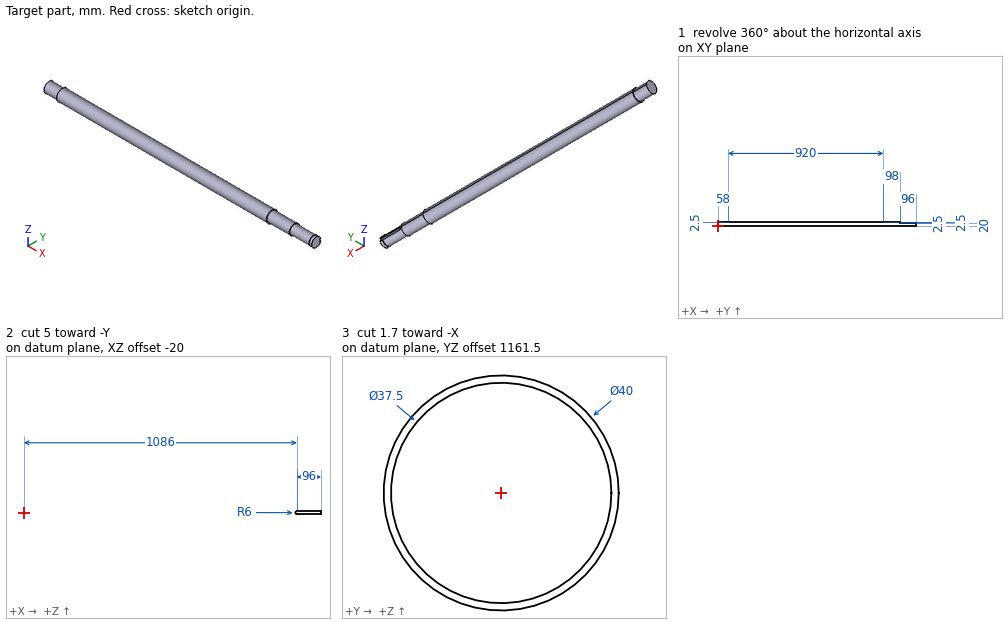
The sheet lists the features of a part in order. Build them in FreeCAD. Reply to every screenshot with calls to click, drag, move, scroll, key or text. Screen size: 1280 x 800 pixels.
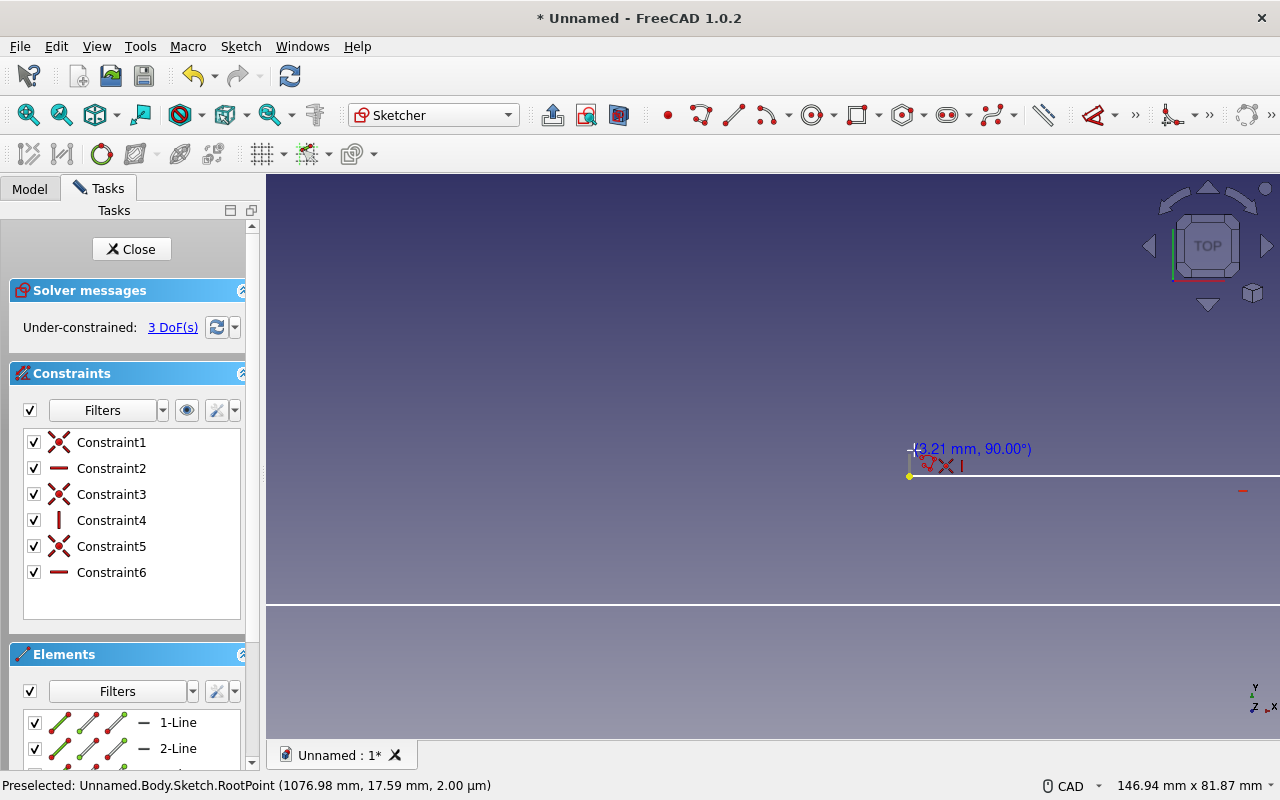
click(910, 450)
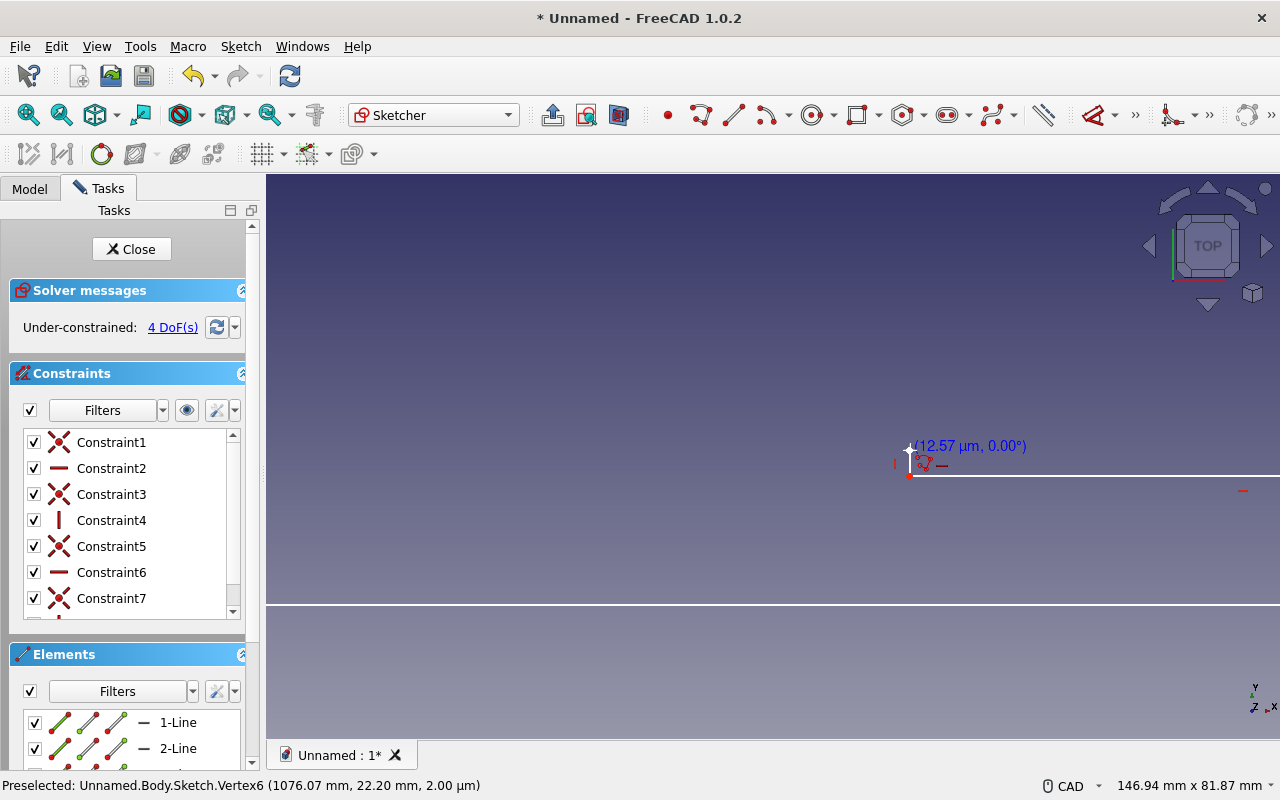
scroll(959, 451, down, 13)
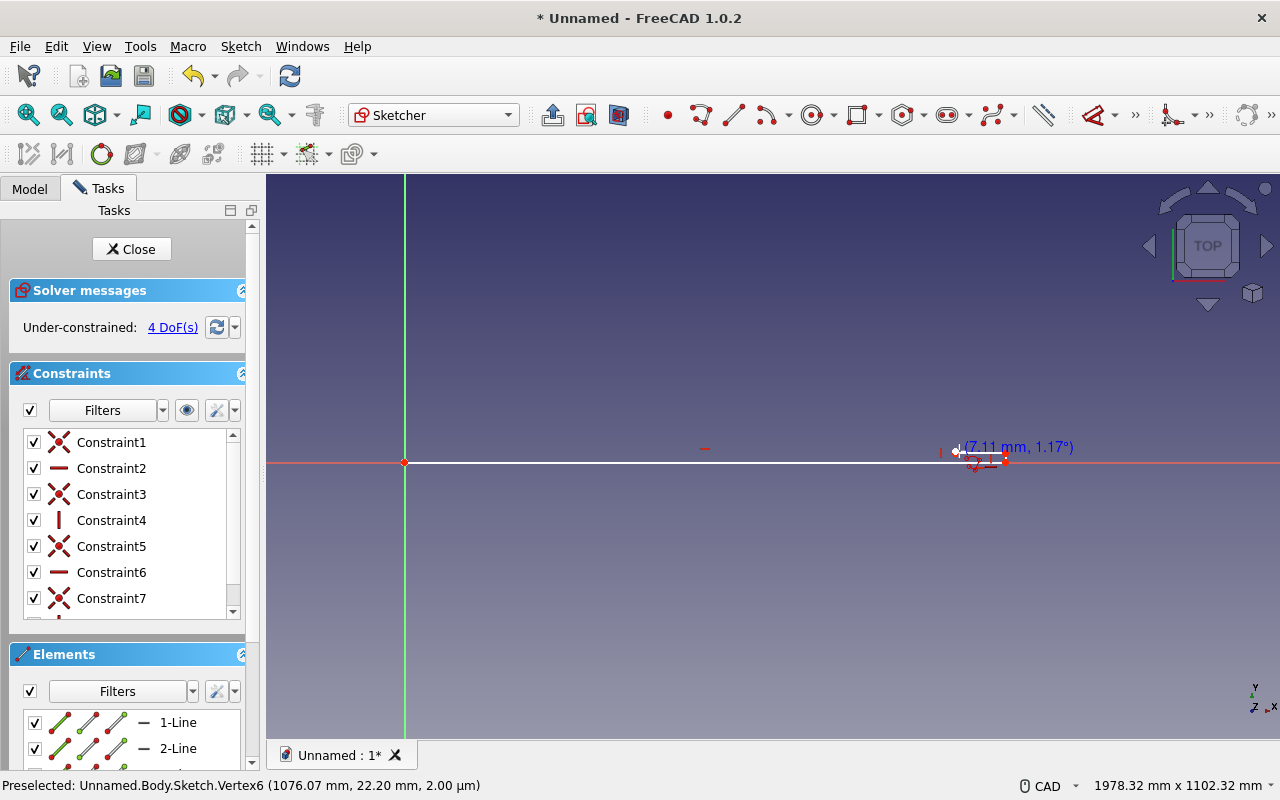
scroll(906, 451, up, 2)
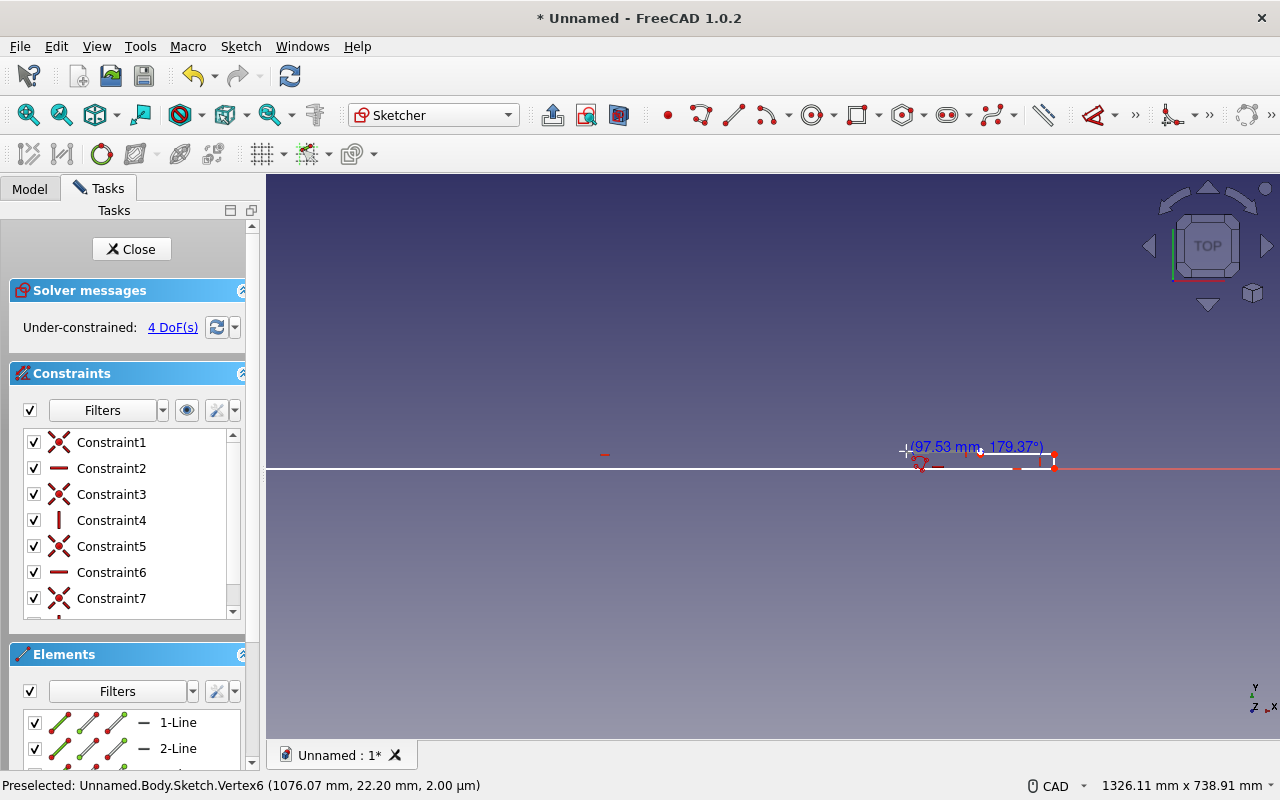
click(905, 451)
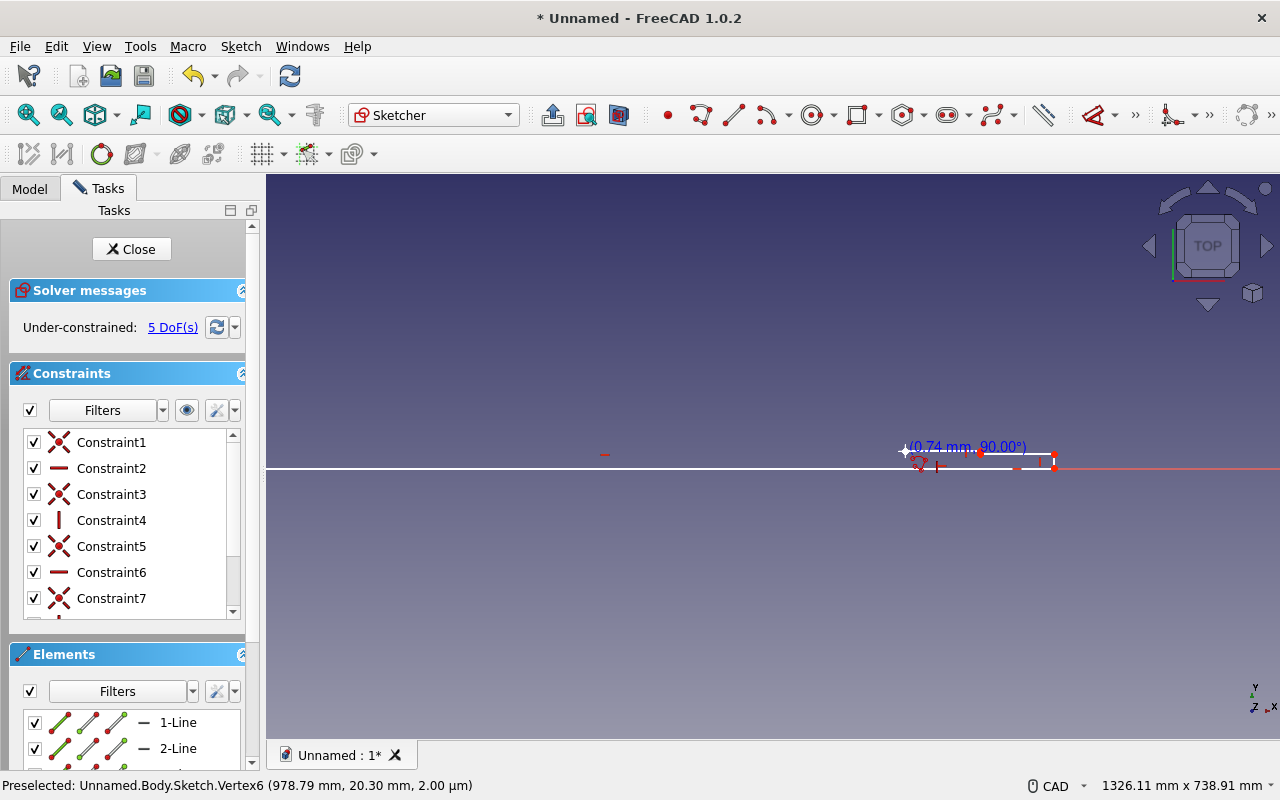
scroll(905, 449, up, 11)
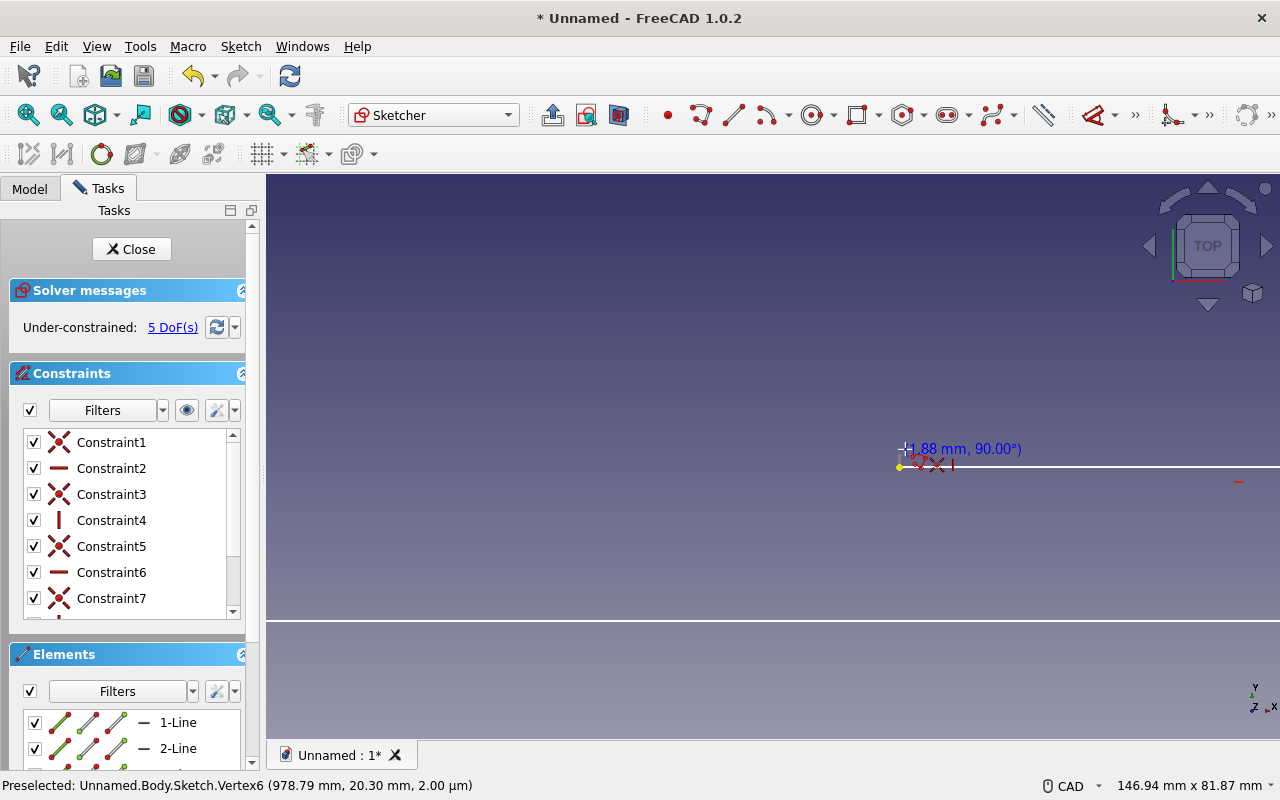
click(900, 449)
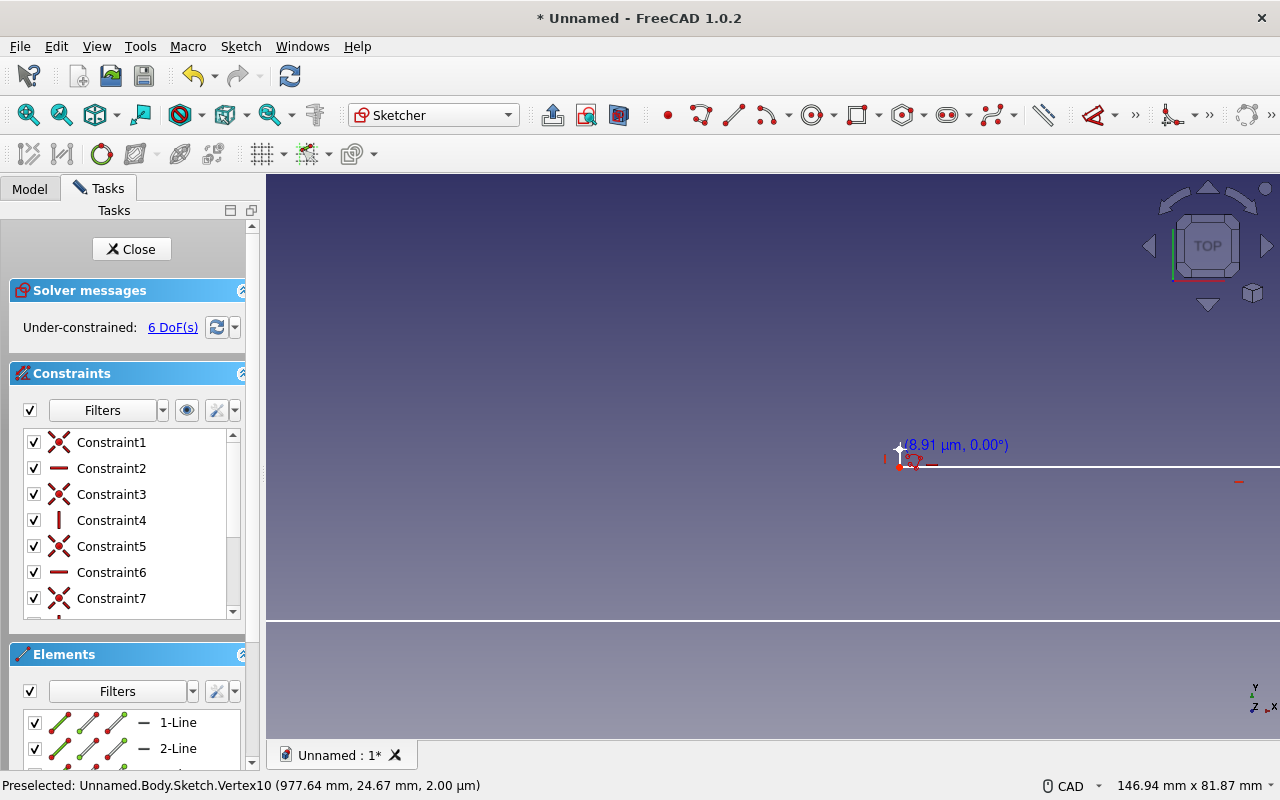
scroll(906, 450, down, 13)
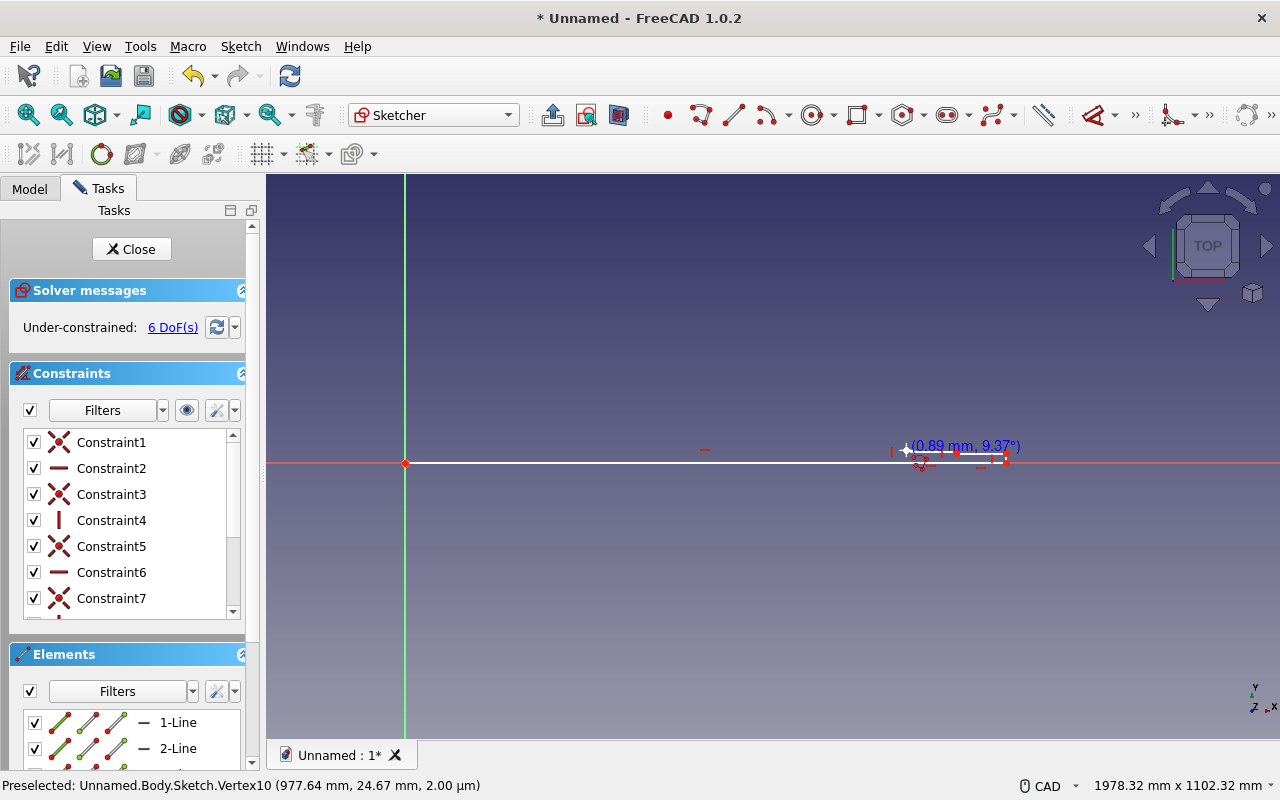
scroll(435, 450, up, 2)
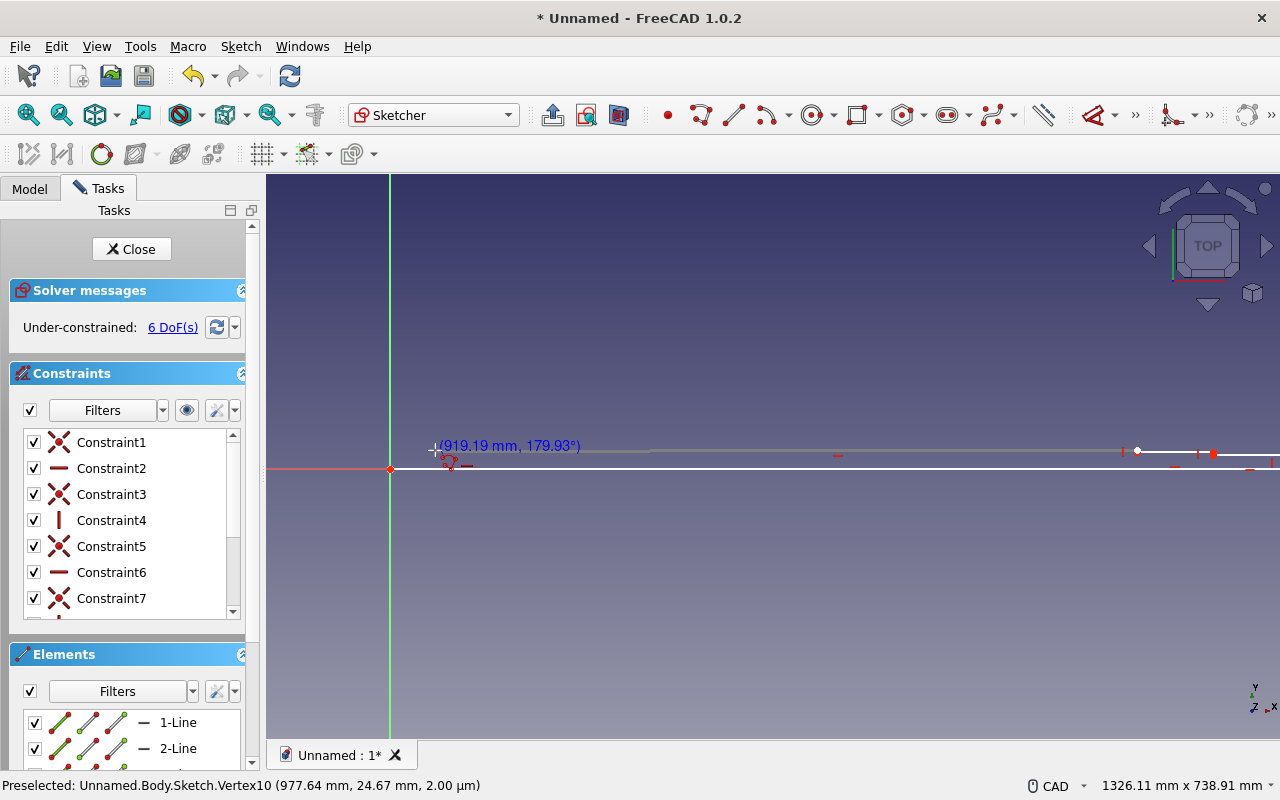
click(435, 450)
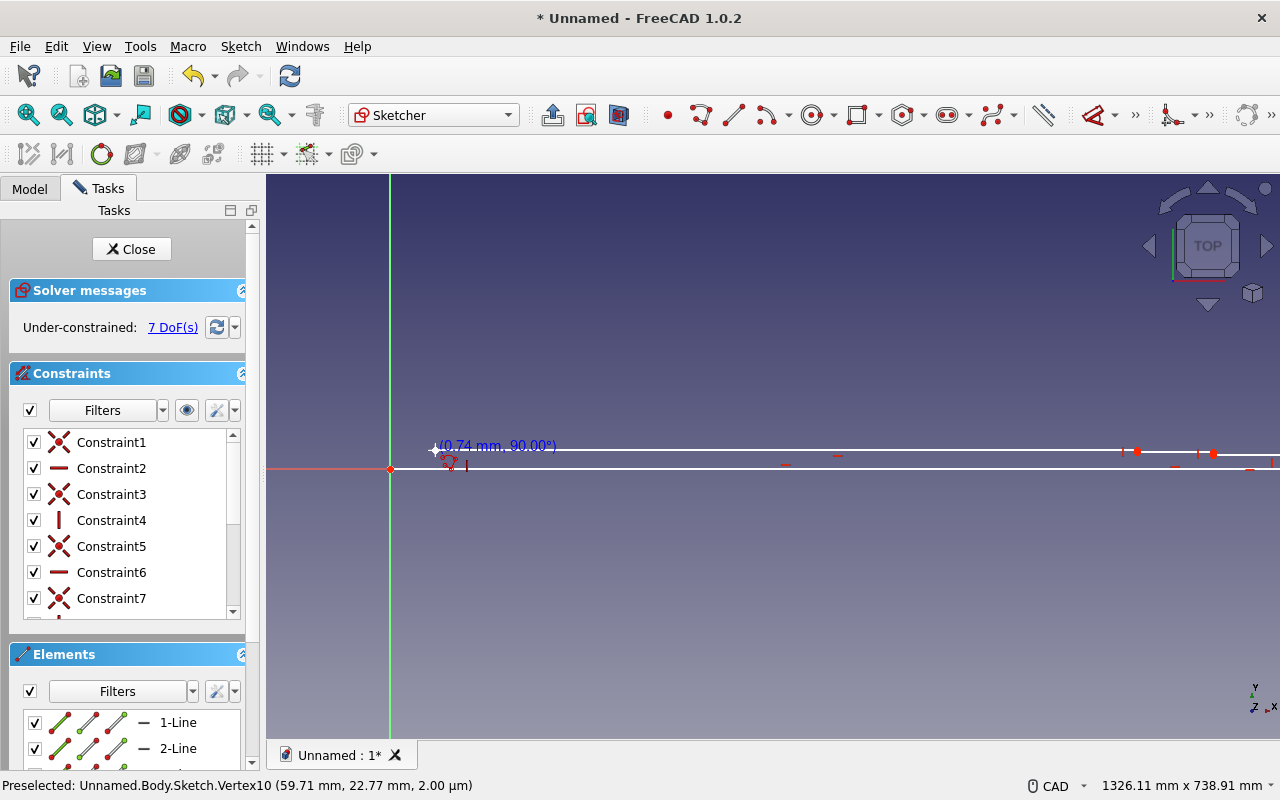
scroll(435, 452, up, 11)